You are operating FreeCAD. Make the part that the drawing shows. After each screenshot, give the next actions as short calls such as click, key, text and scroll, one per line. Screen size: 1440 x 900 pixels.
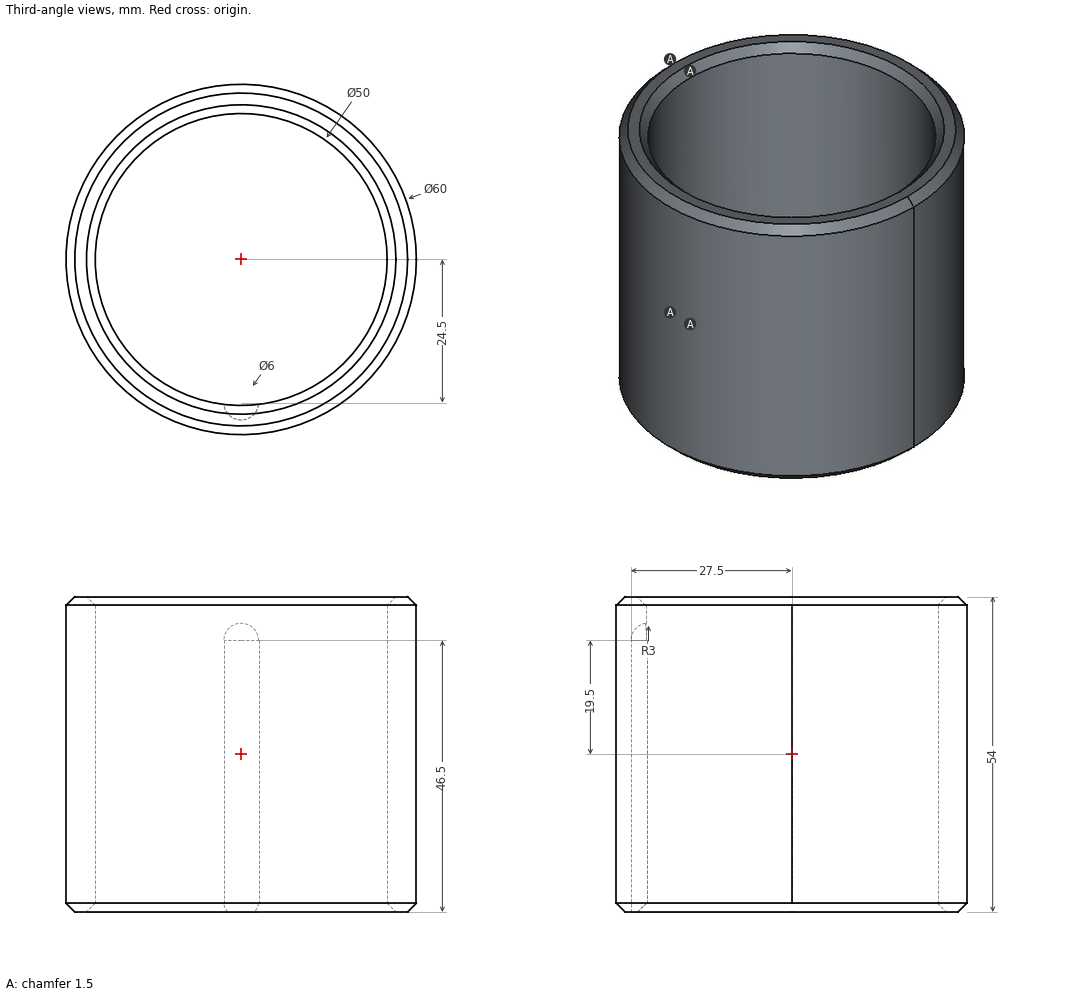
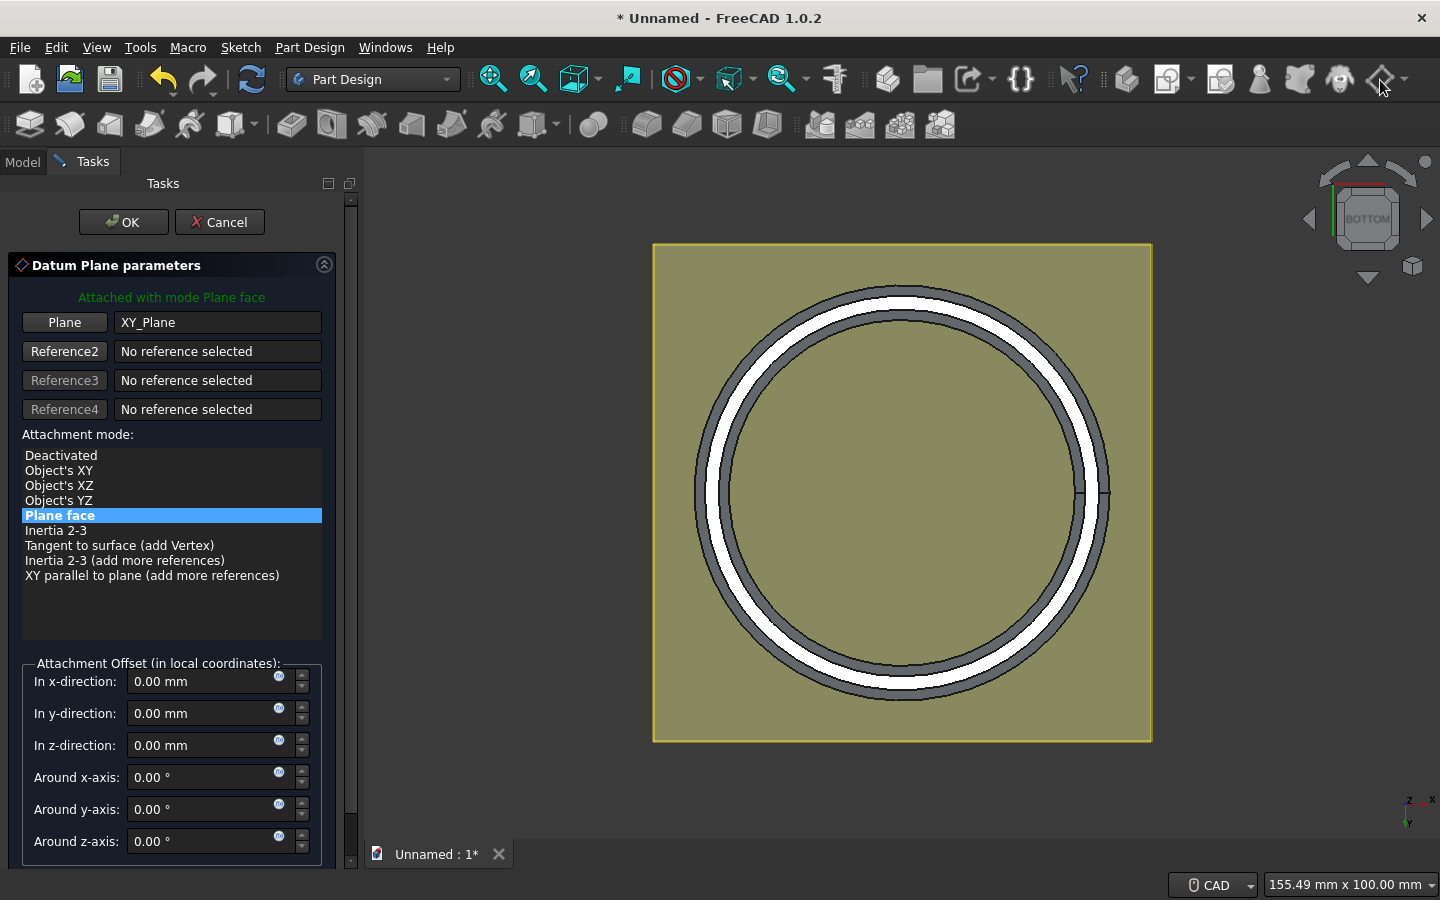
triple_click(210, 745)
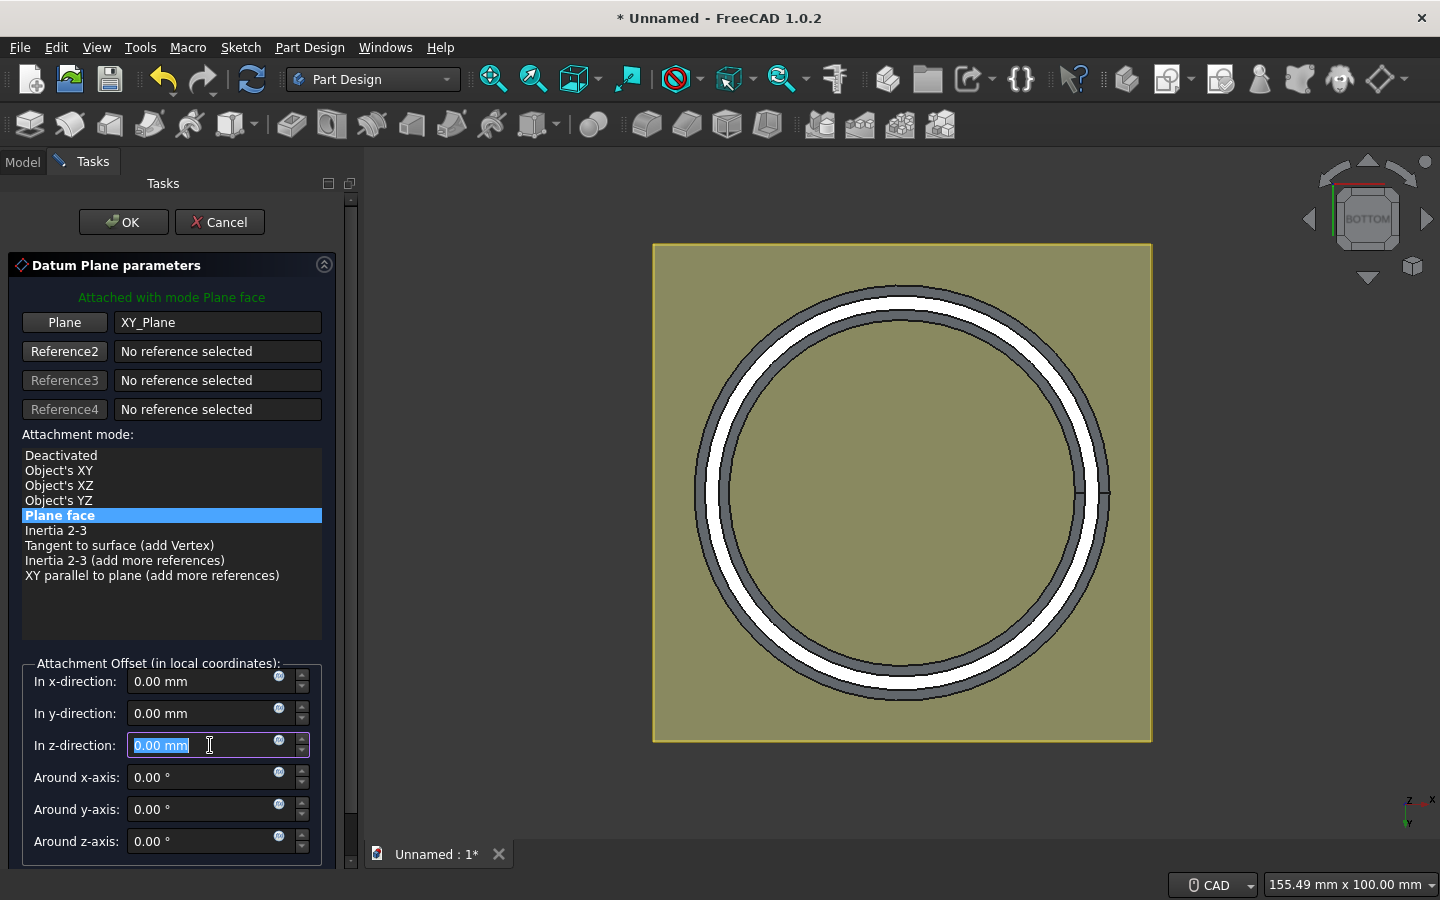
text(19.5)
key(Tab)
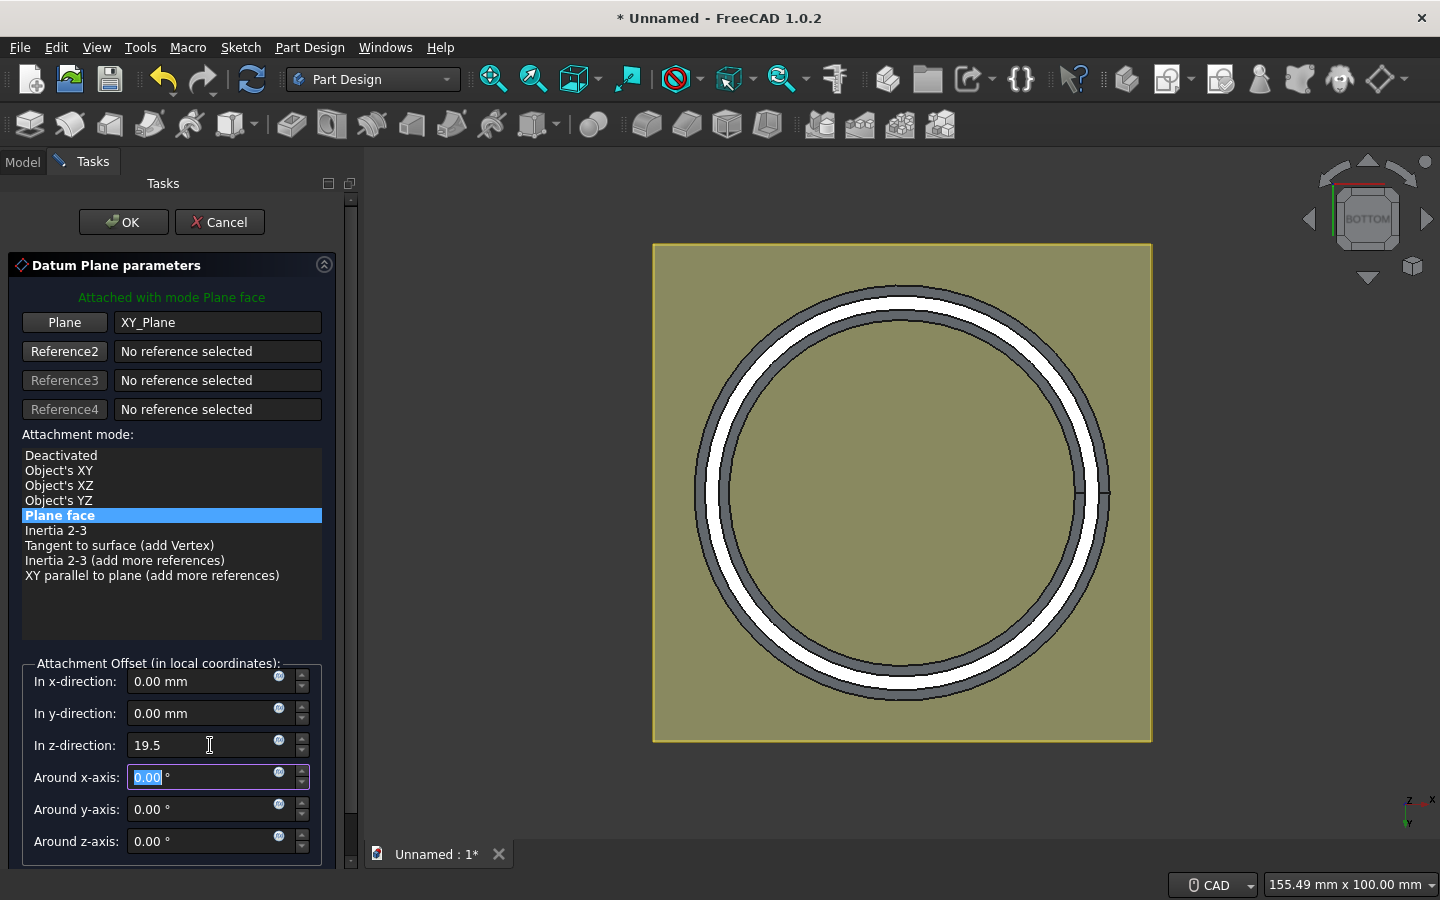
click(124, 222)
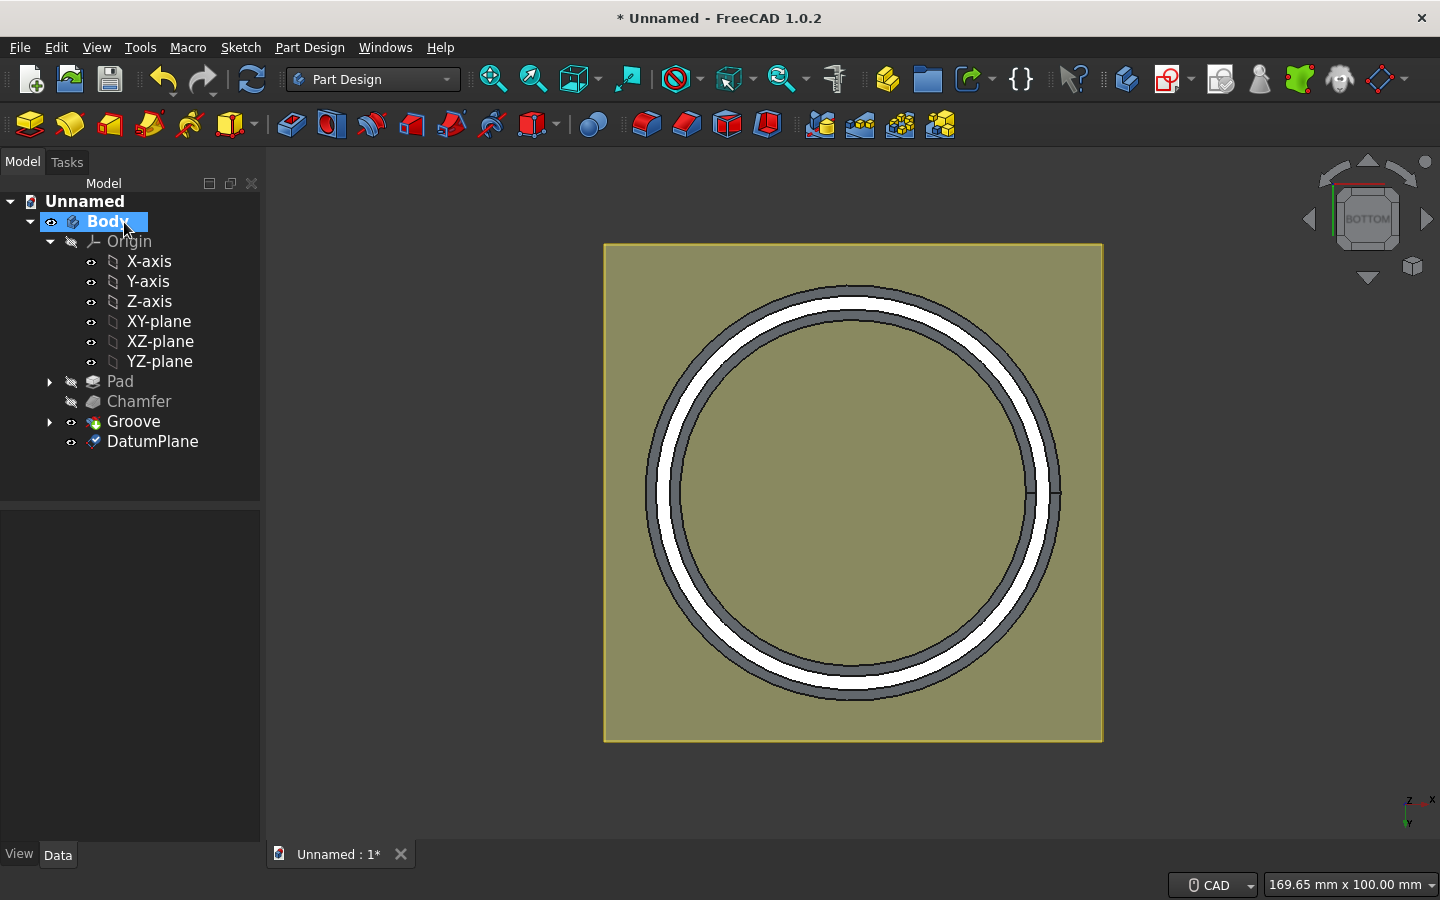
click(116, 442)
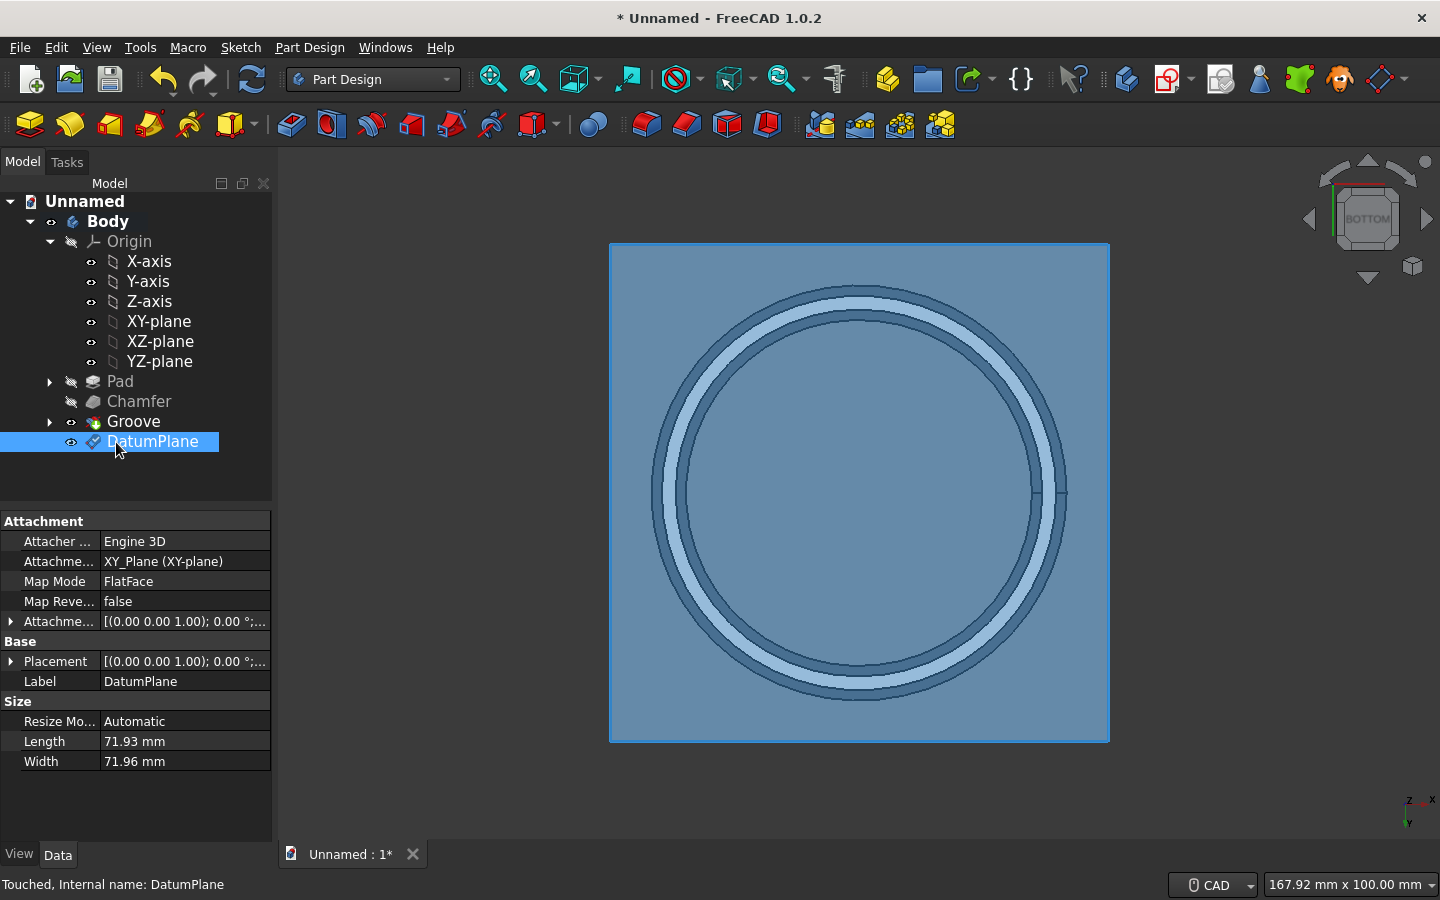
click(1168, 80)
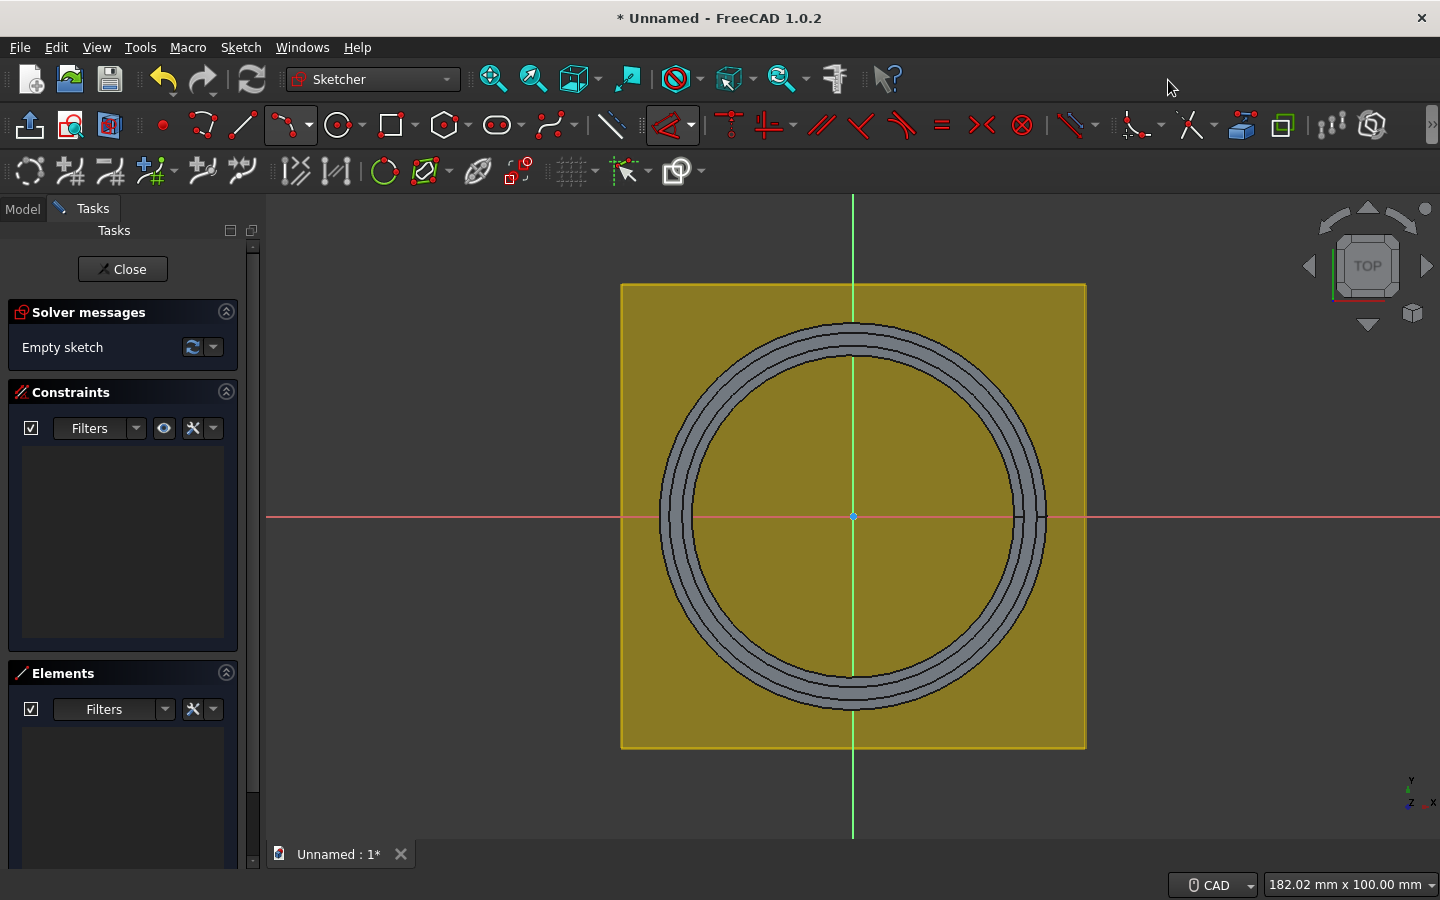
click(110, 126)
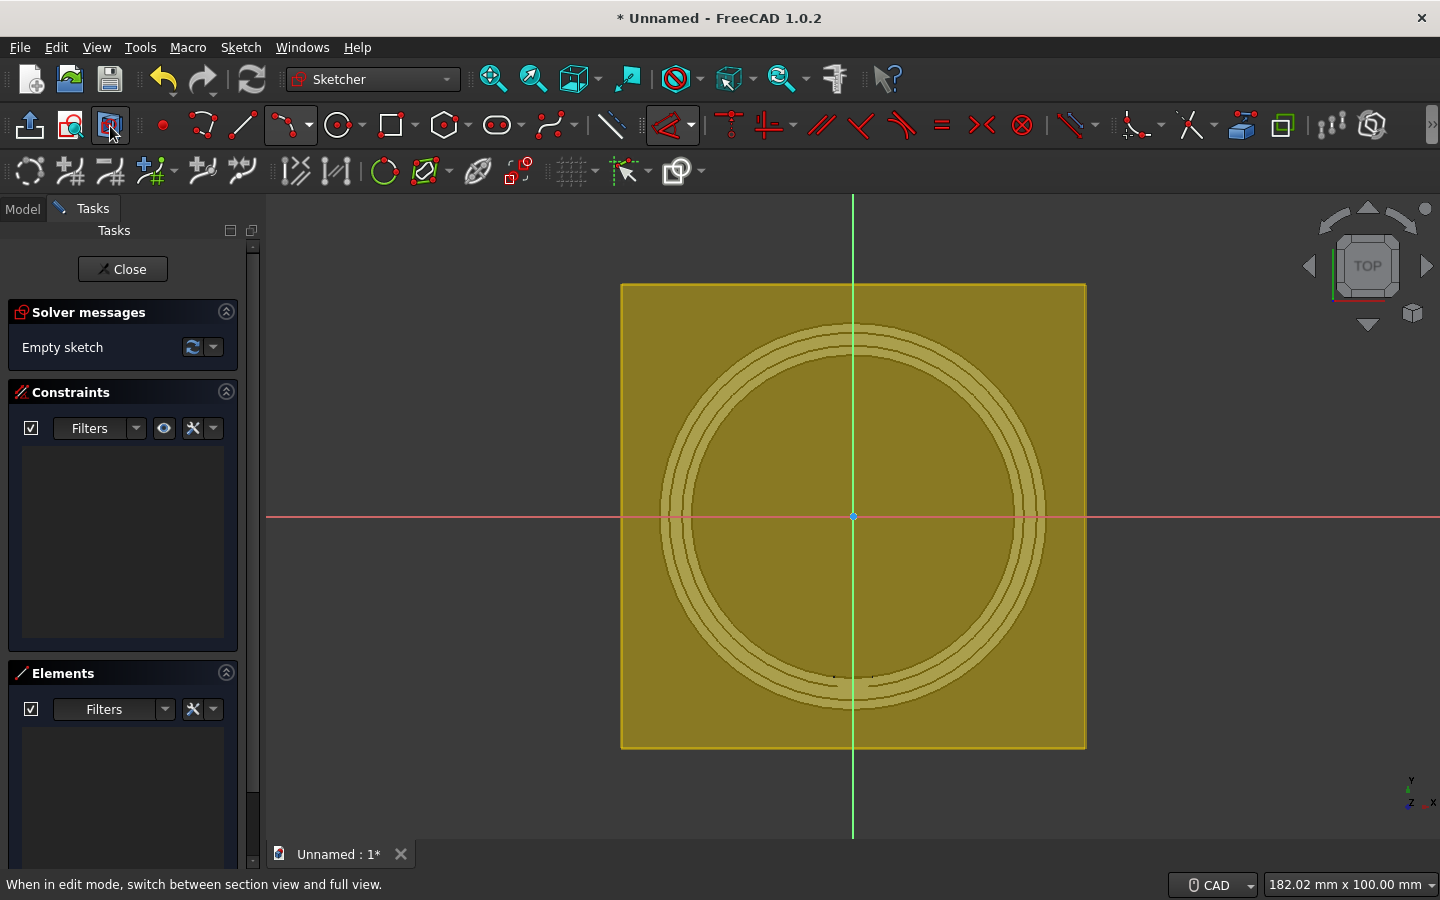
scroll(860, 690, up, 12)